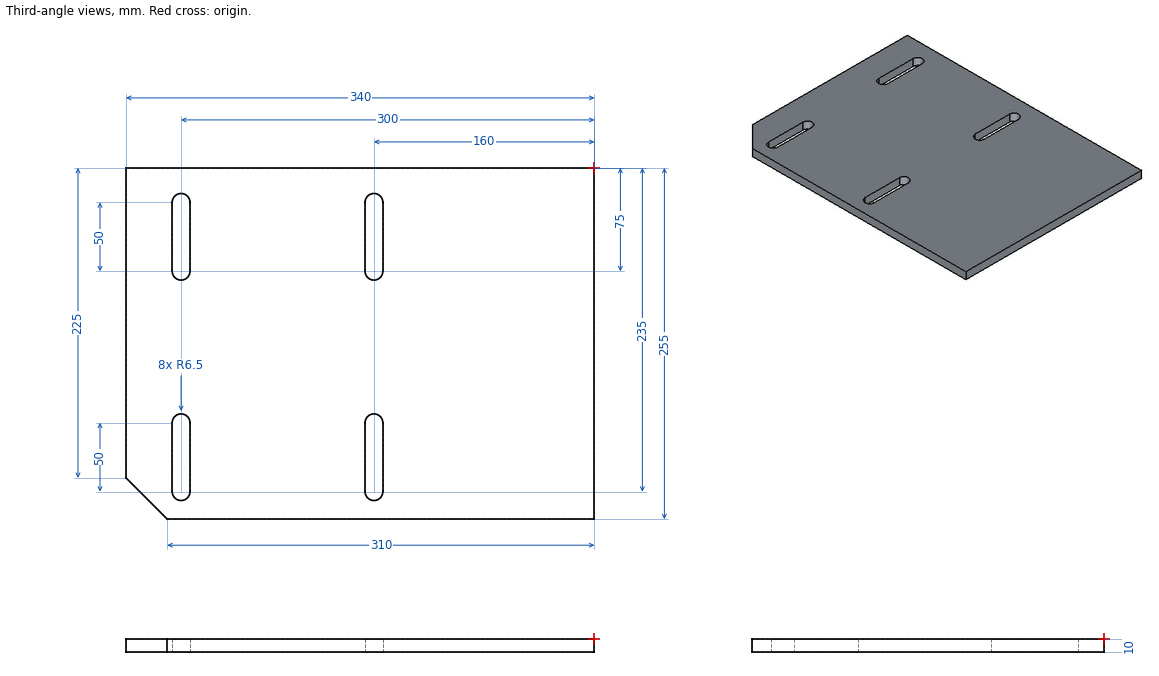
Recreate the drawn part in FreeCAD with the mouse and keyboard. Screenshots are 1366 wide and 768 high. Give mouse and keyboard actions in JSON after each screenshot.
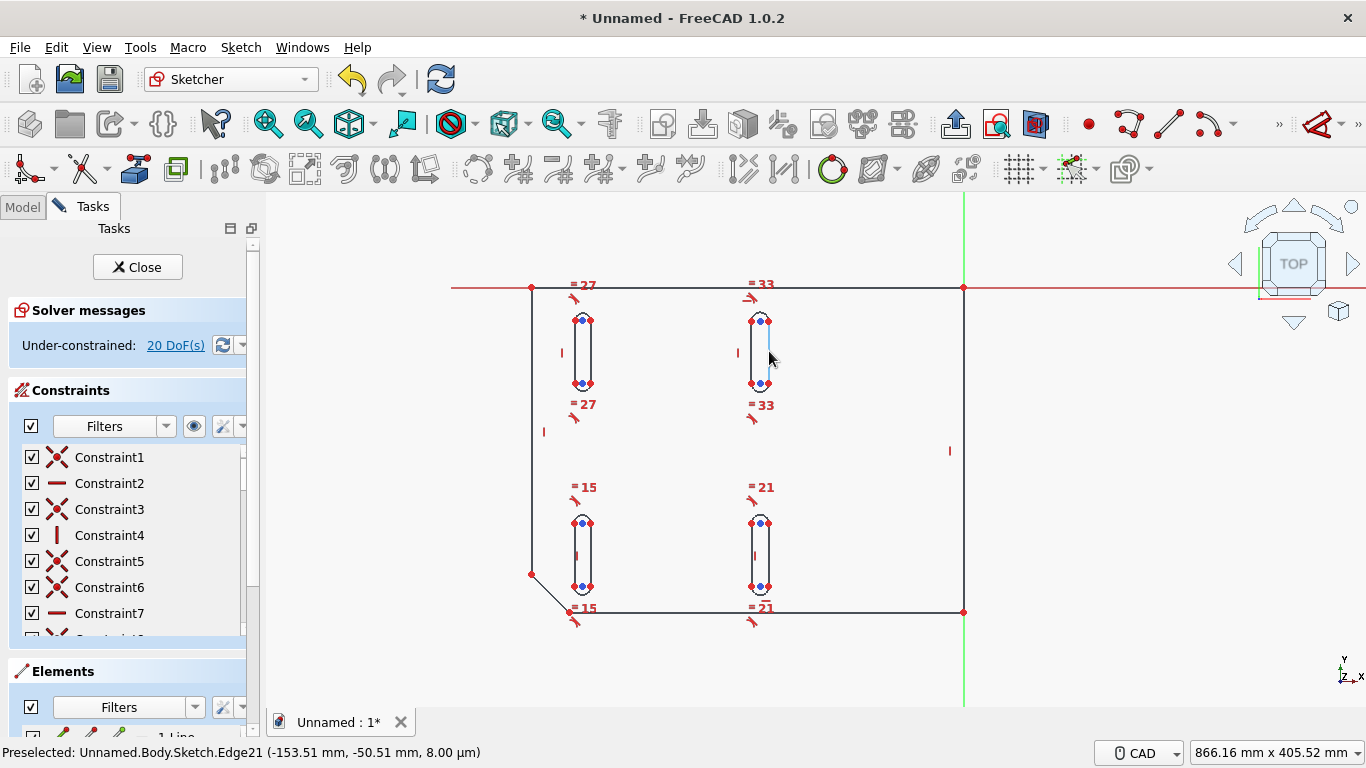
{"action": "scroll", "coordinate": [578, 593], "scroll_direction": "up", "scroll_amount": 4}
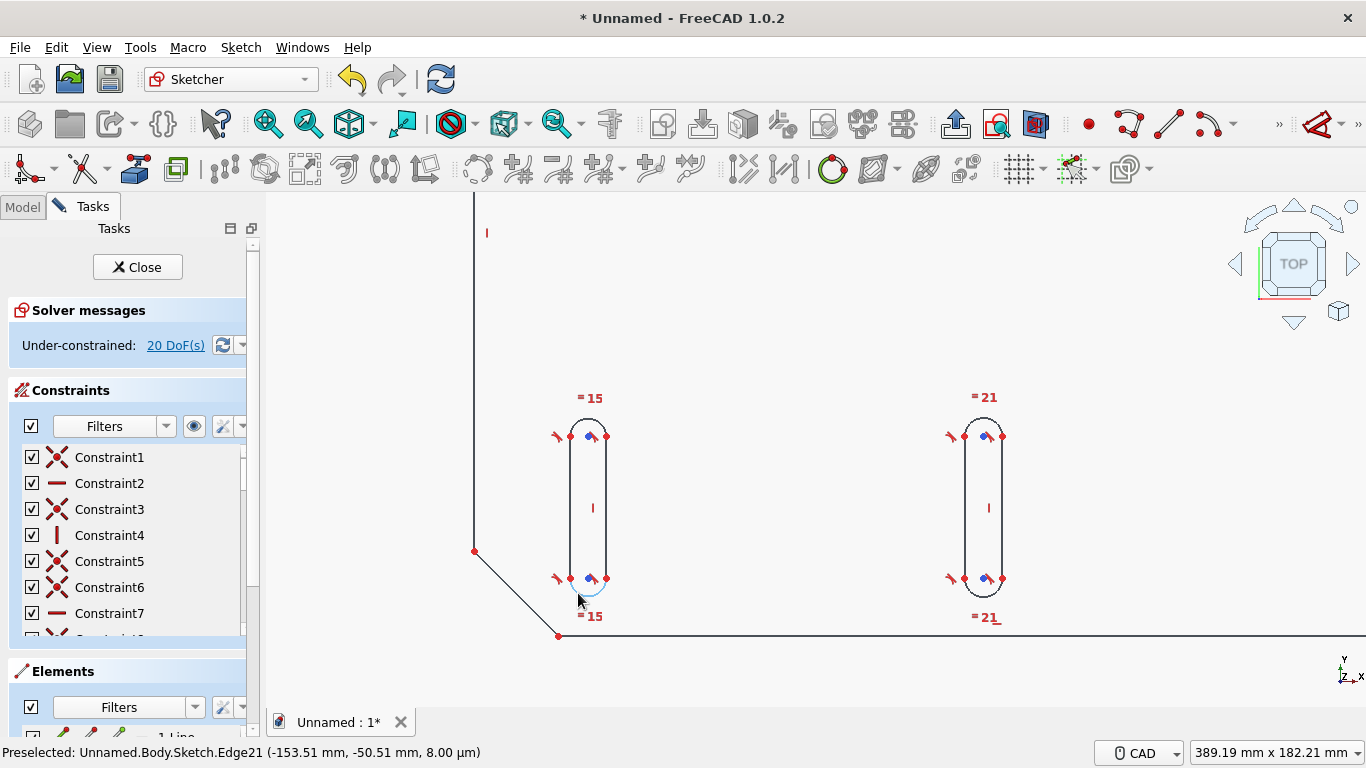
{"action": "left_click", "coordinate": [577, 593]}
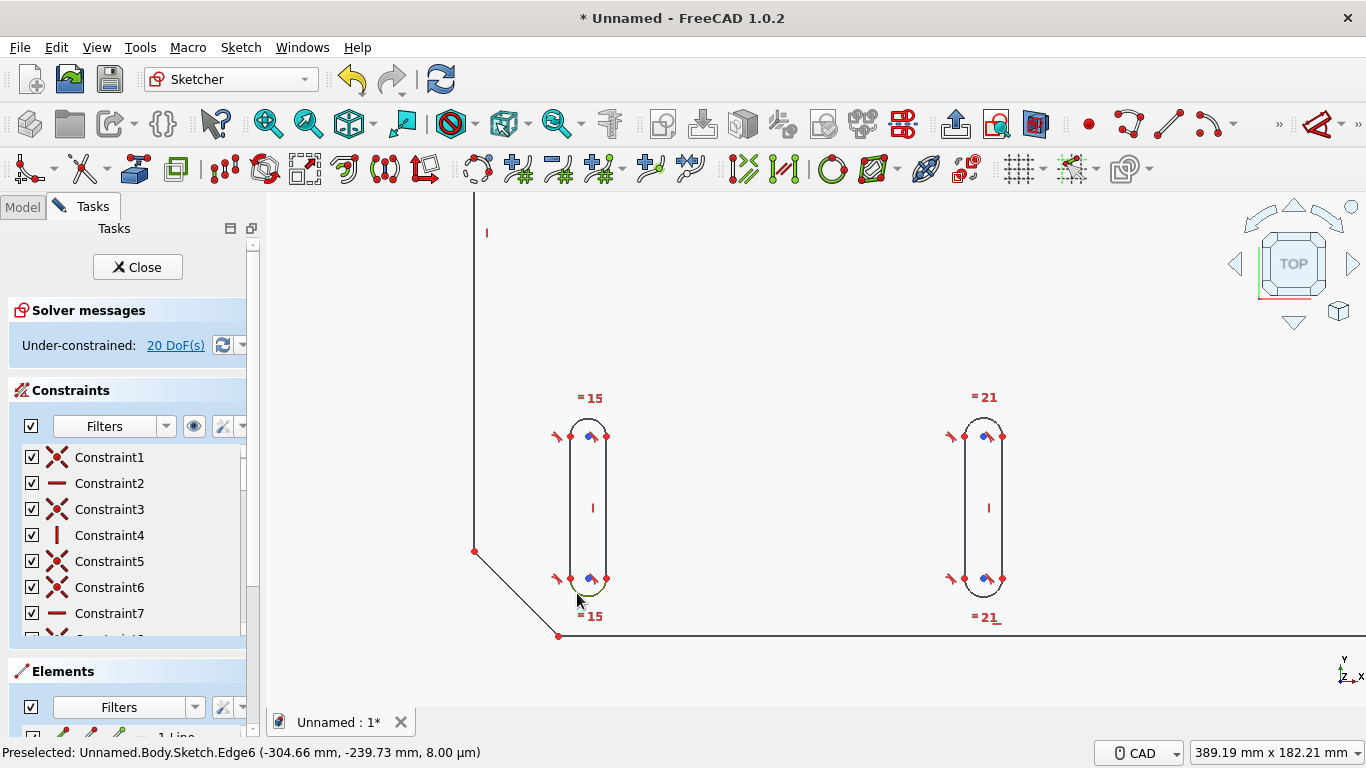
{"action": "left_click", "coordinate": [973, 593]}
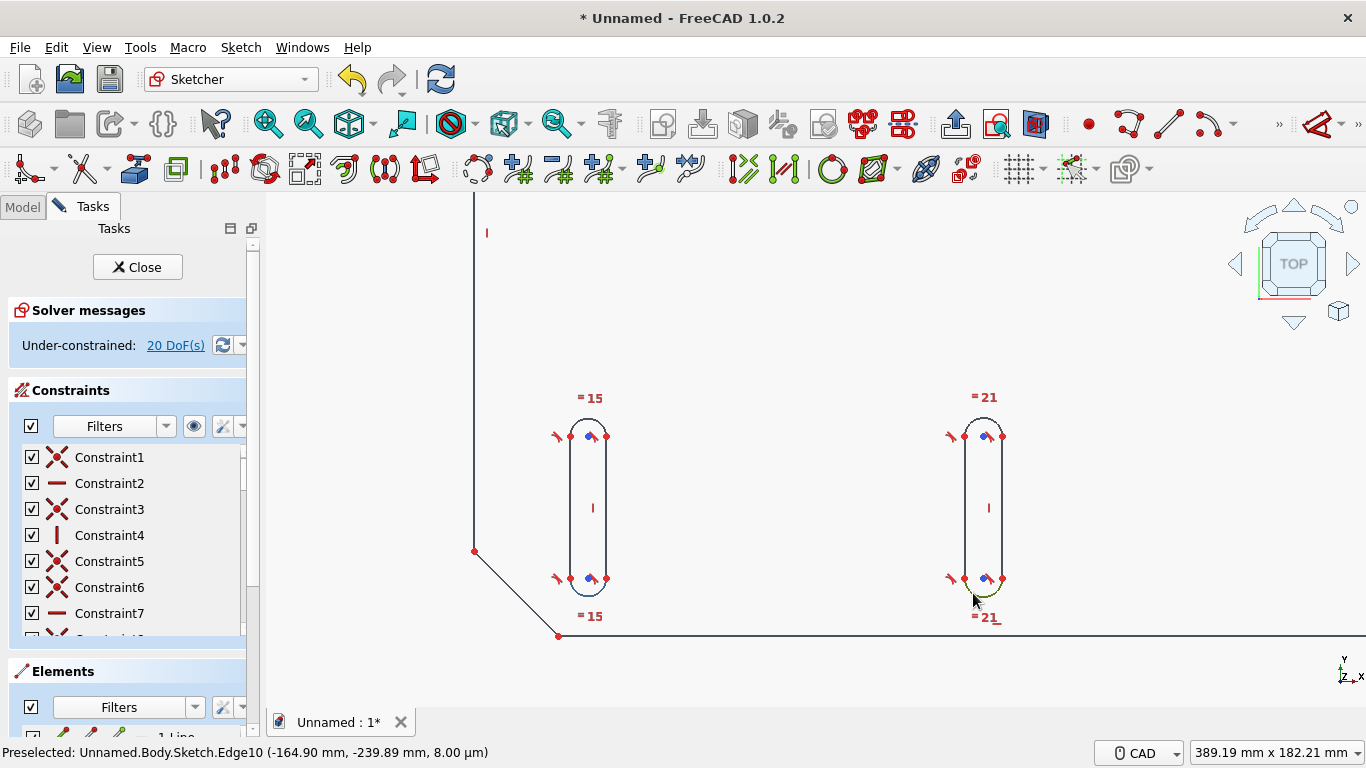
{"action": "scroll", "coordinate": [578, 593], "scroll_direction": "down", "scroll_amount": 4}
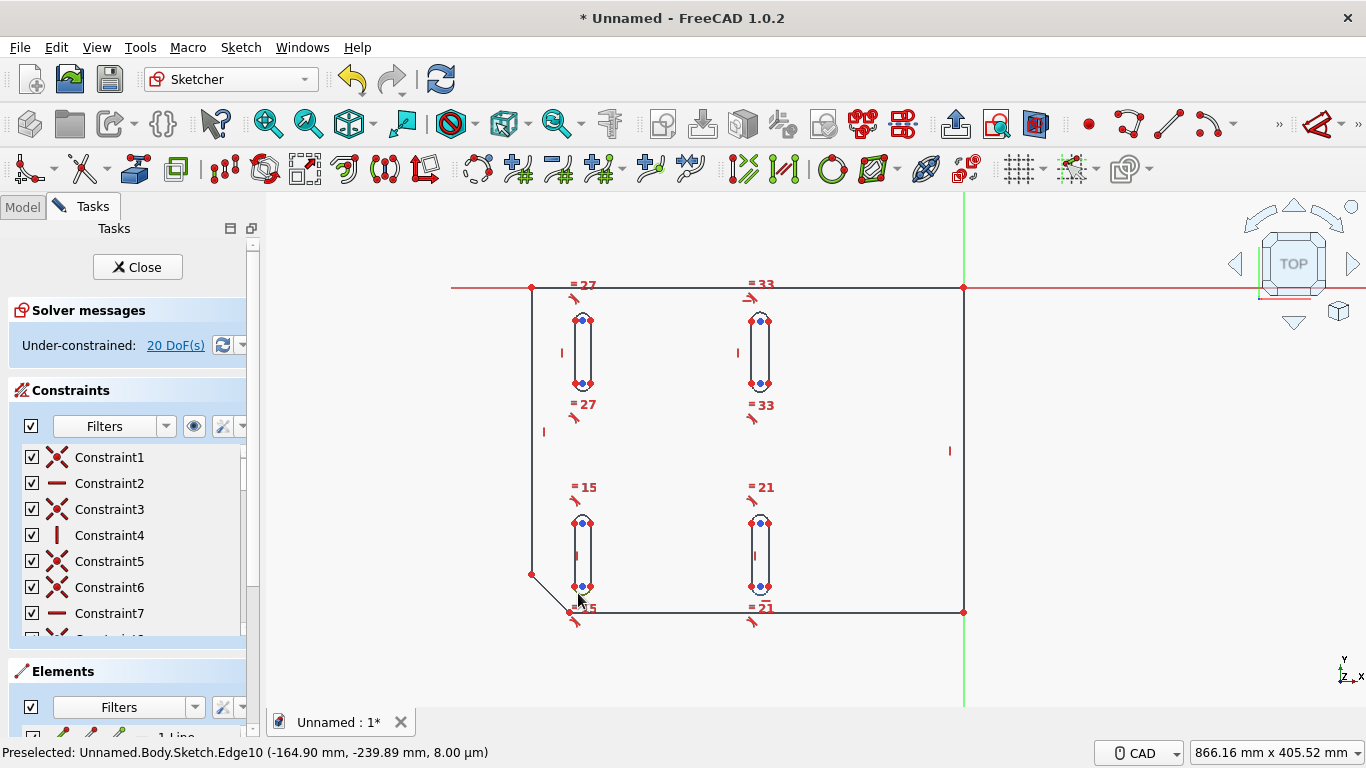
{"action": "scroll", "coordinate": [578, 390], "scroll_direction": "up", "scroll_amount": 4}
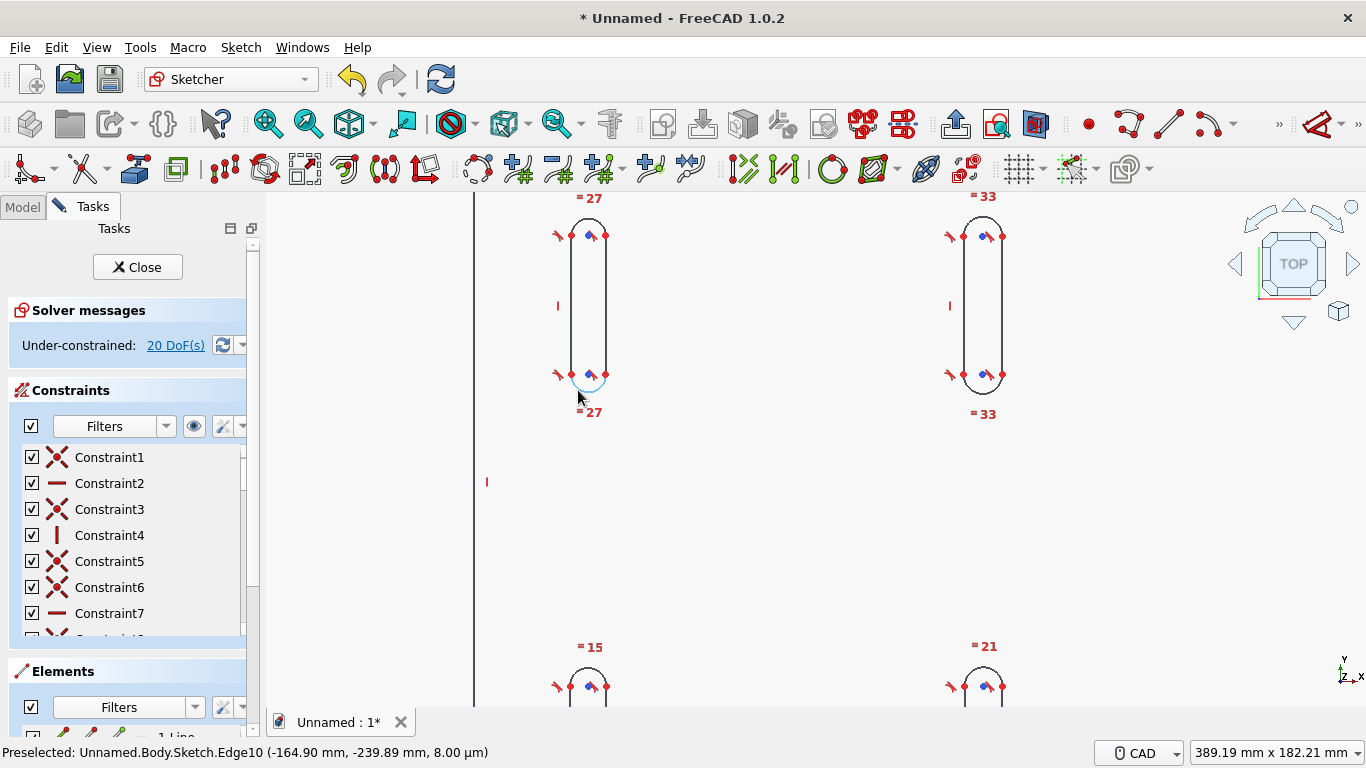
{"action": "left_click", "coordinate": [578, 389]}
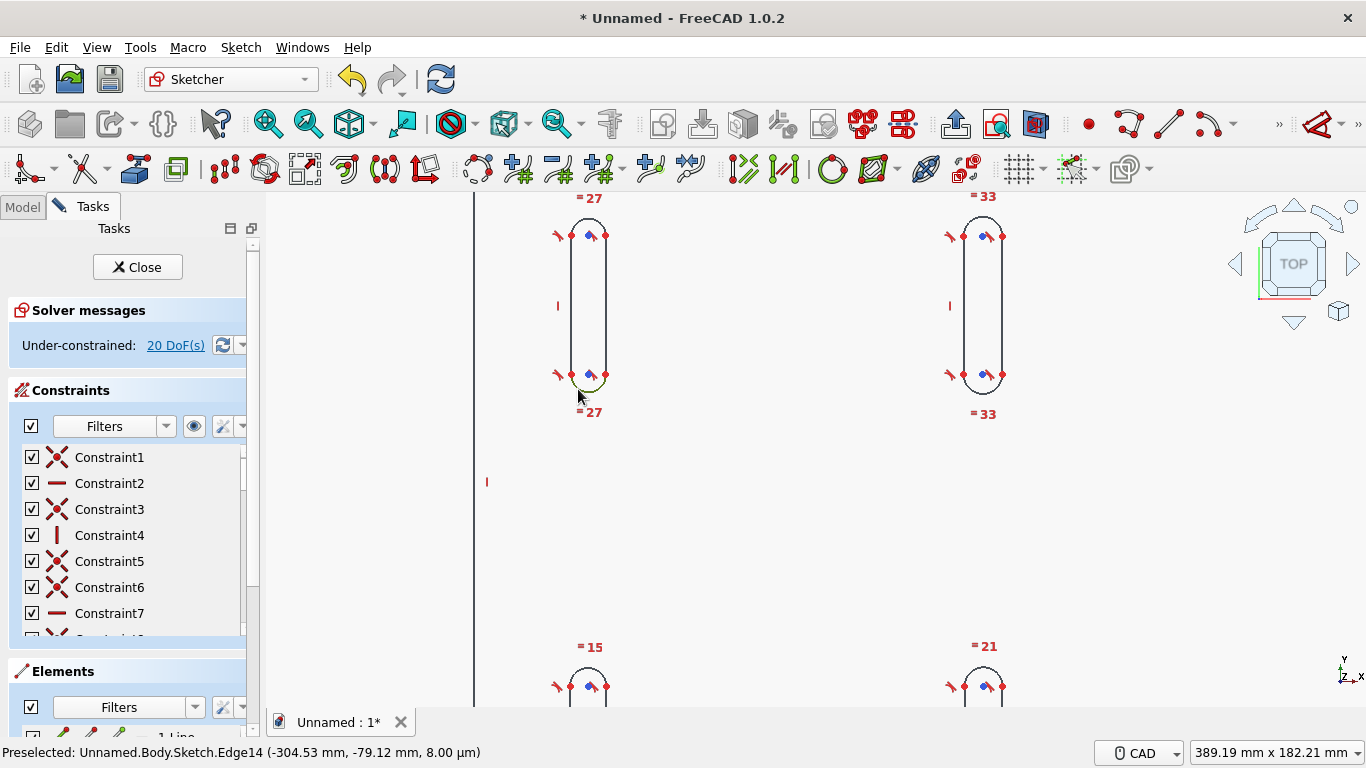
{"action": "left_click", "coordinate": [972, 390]}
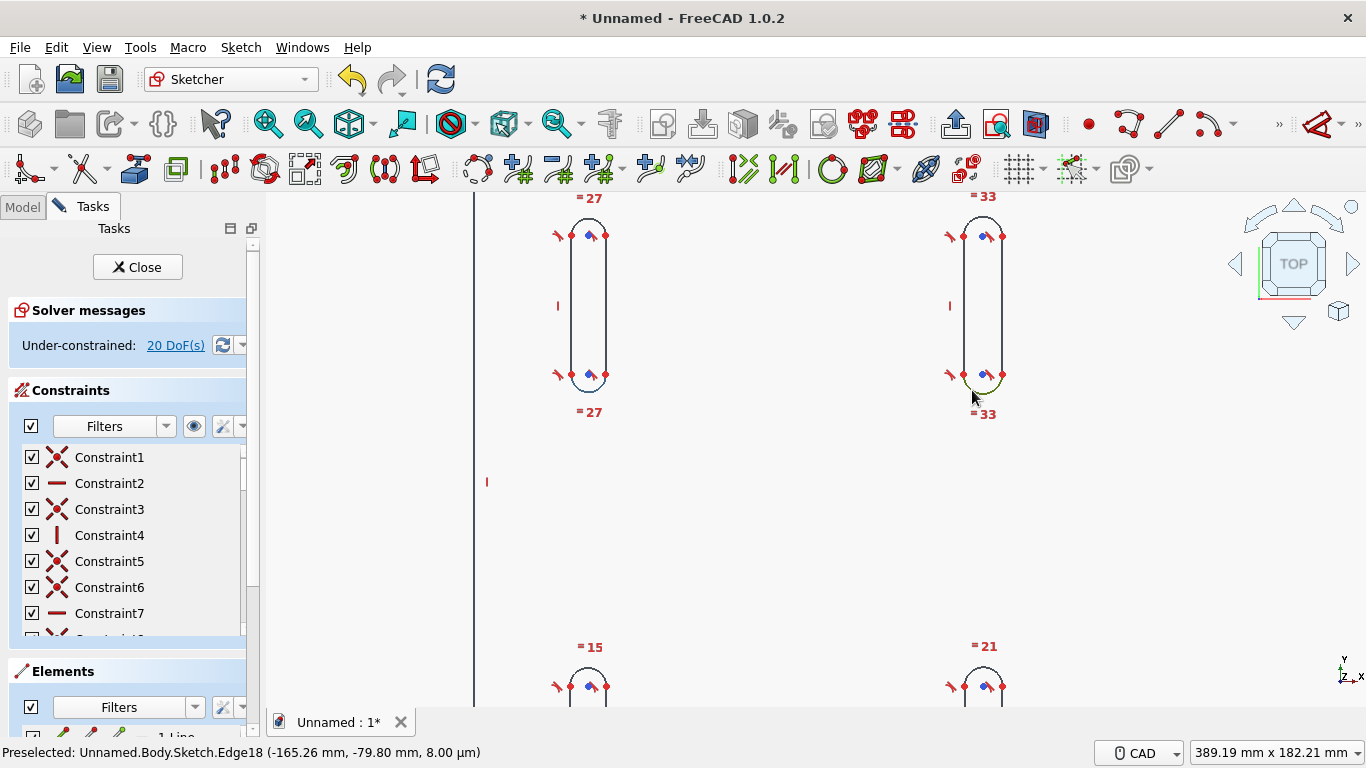
{"action": "key", "text": "e"}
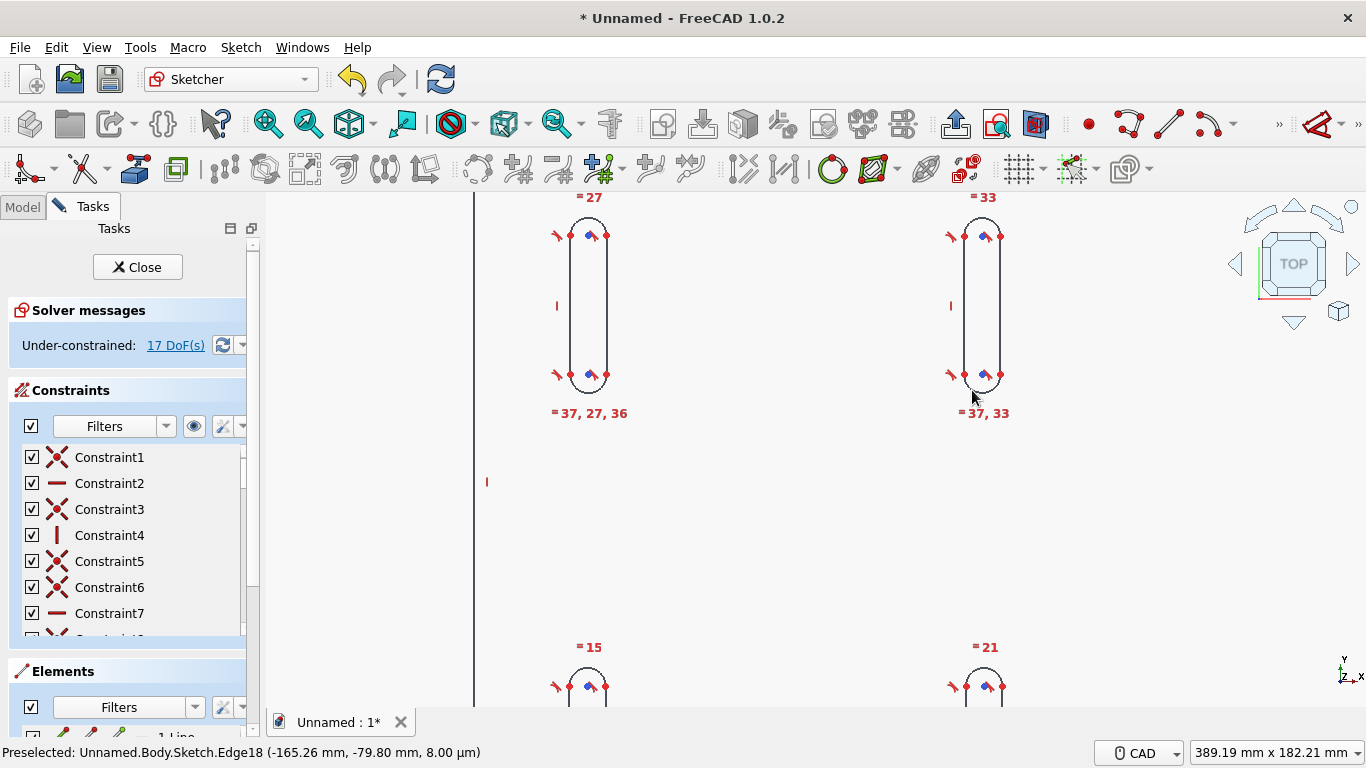
{"action": "key", "text": "d"}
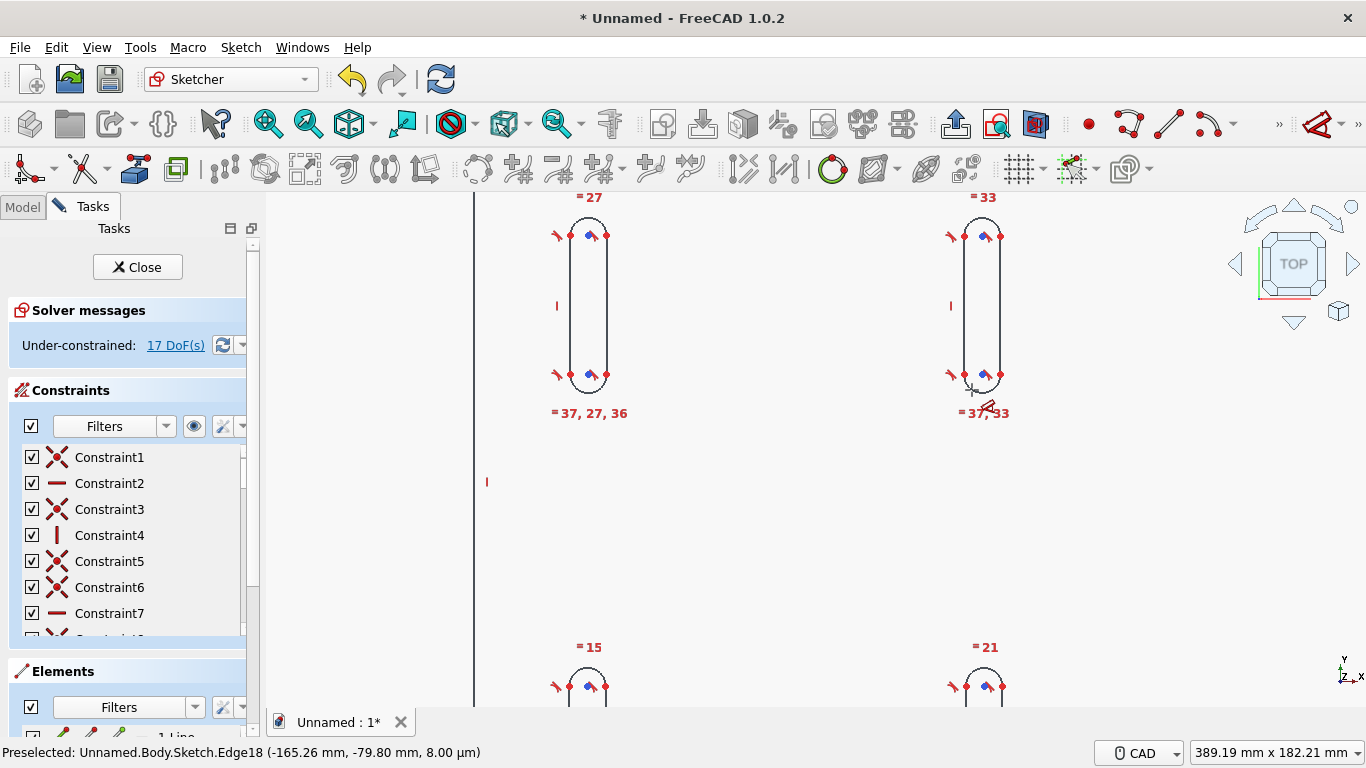
{"action": "scroll", "coordinate": [578, 390], "scroll_direction": "down", "scroll_amount": 4}